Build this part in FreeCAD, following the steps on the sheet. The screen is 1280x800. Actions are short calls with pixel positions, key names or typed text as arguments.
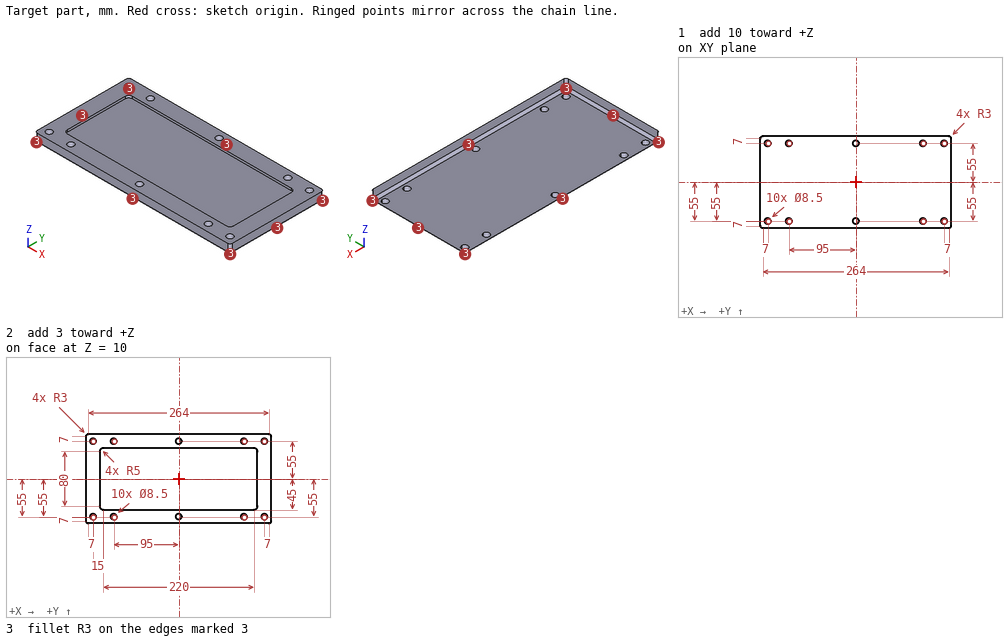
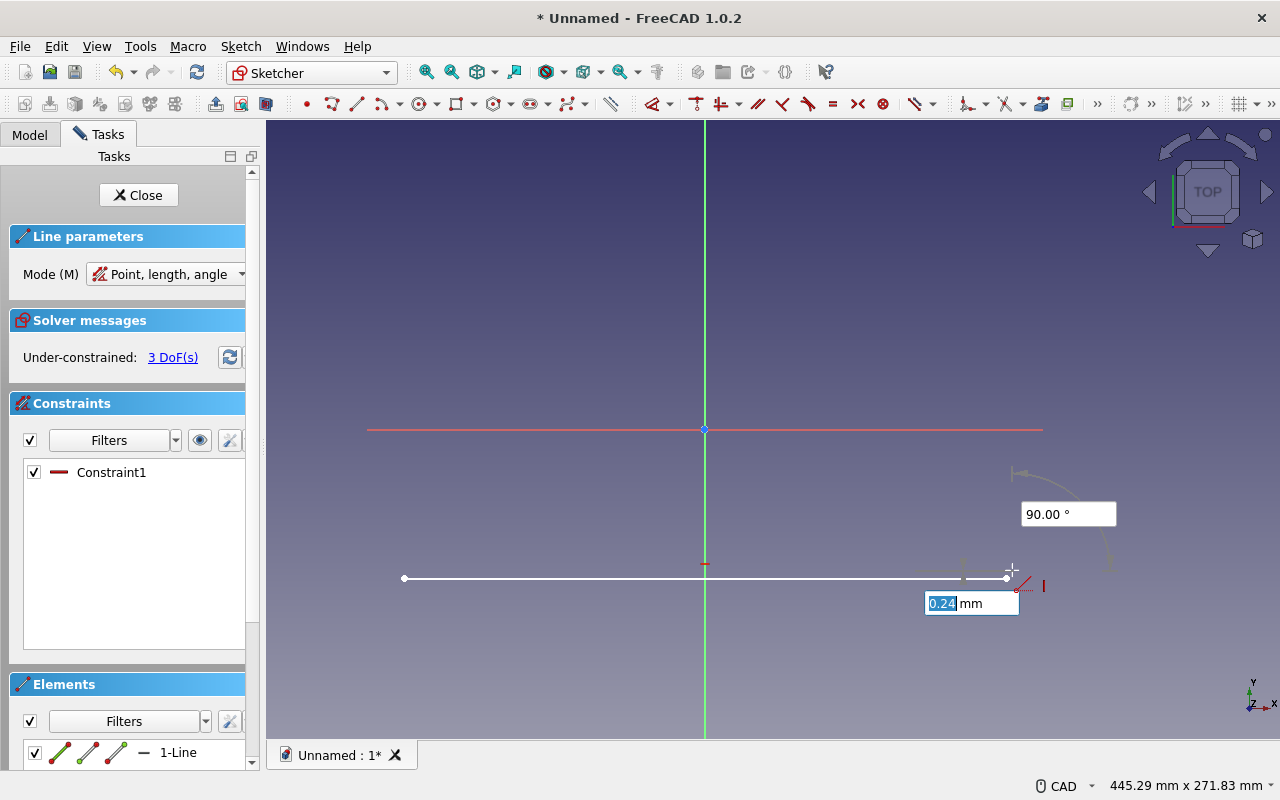
click(1012, 288)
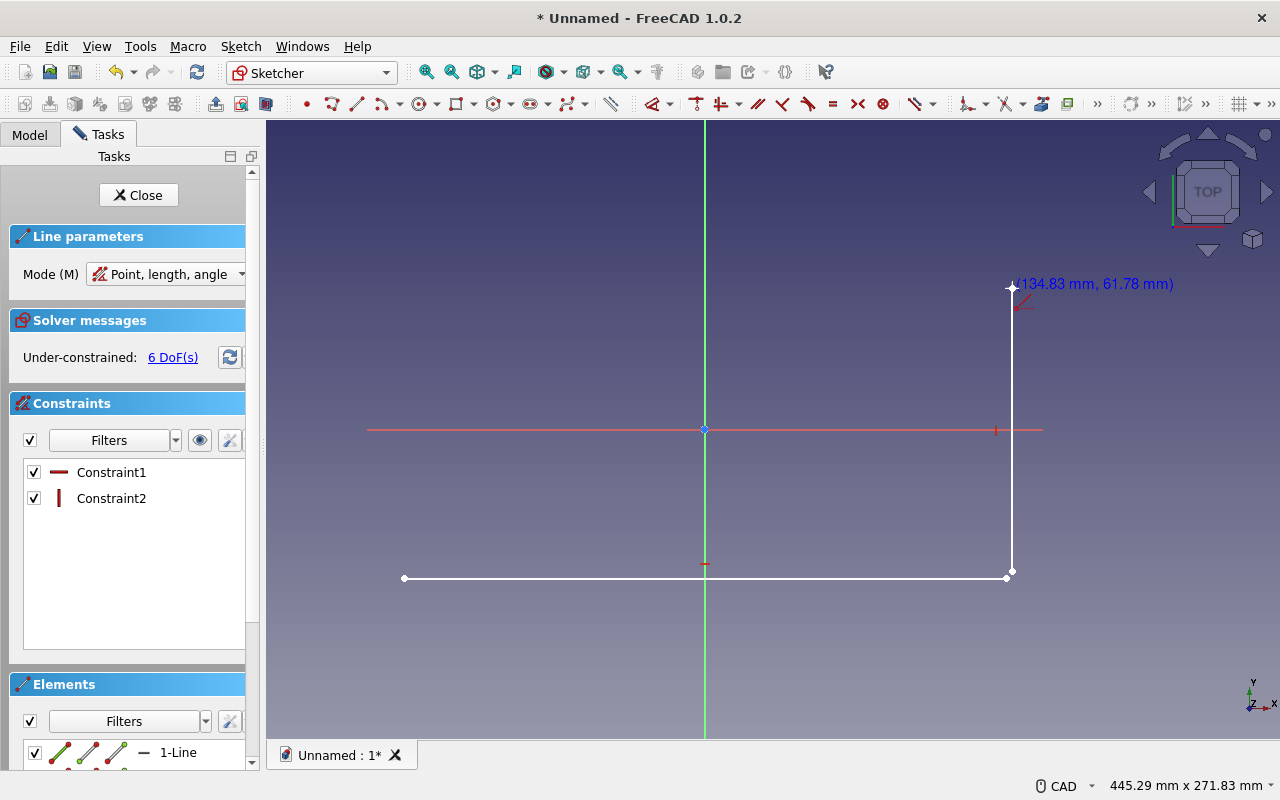
scroll(1006, 282, up, 3)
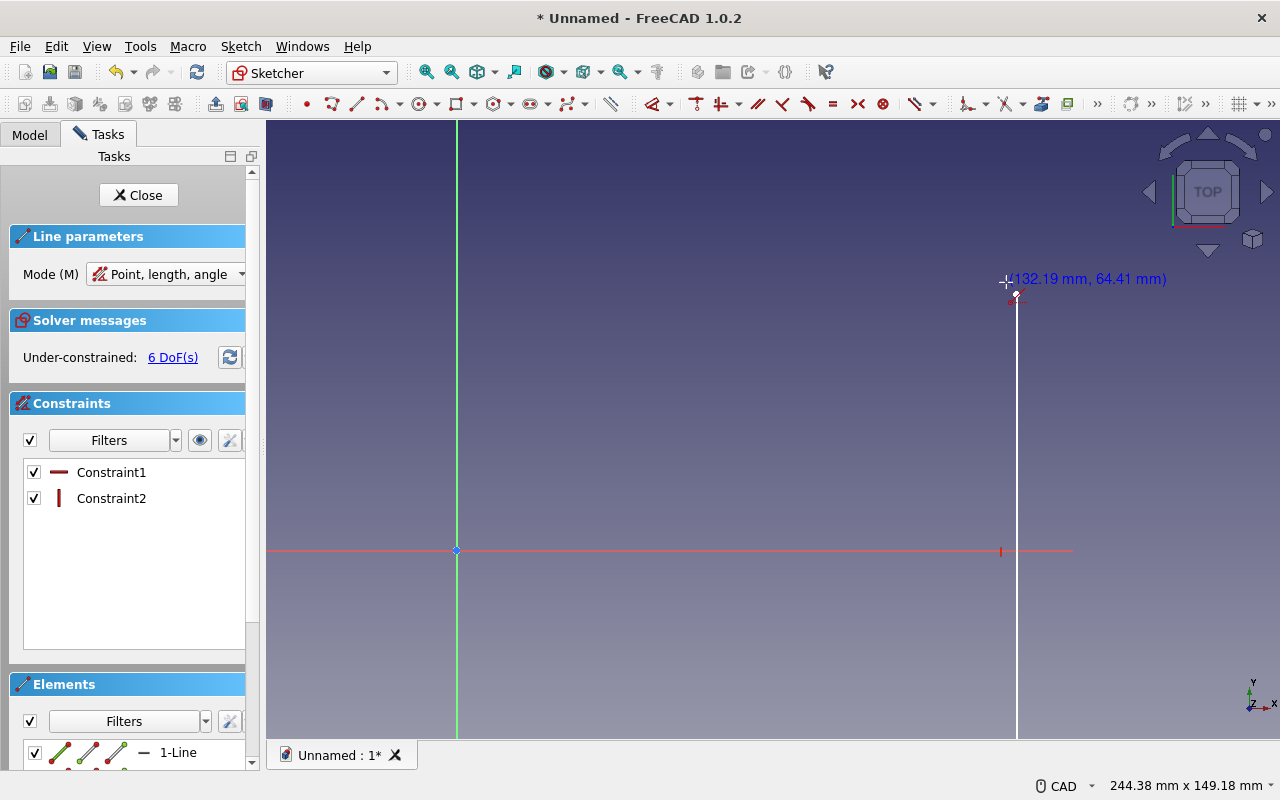
click(1005, 281)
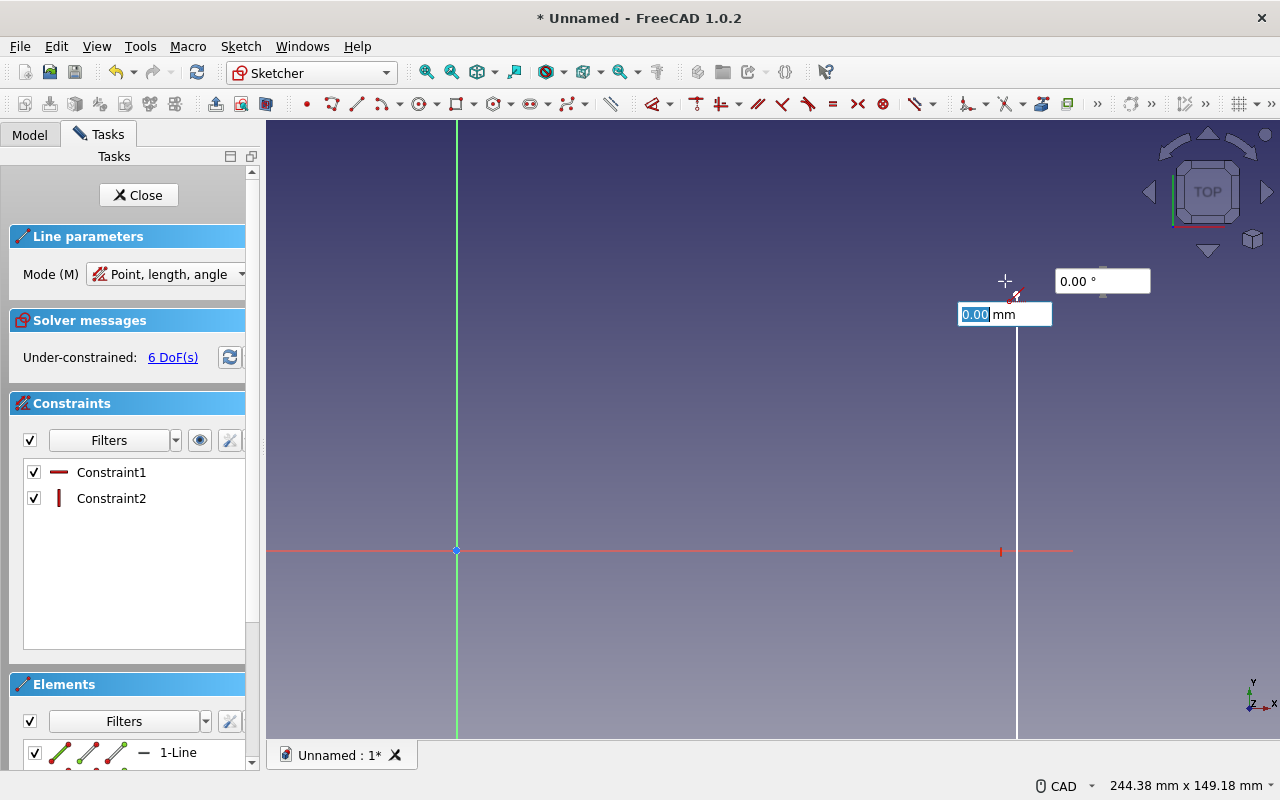
scroll(1006, 282, down, 3)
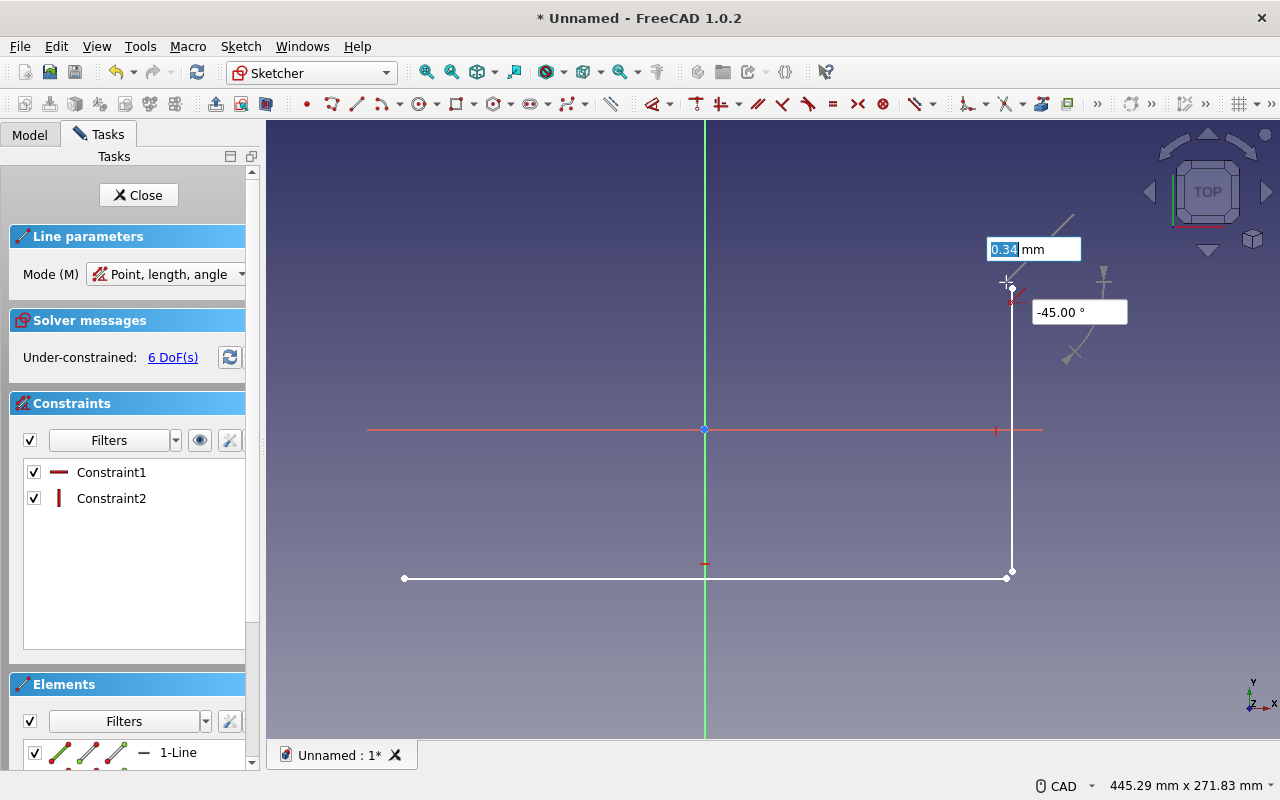
click(404, 282)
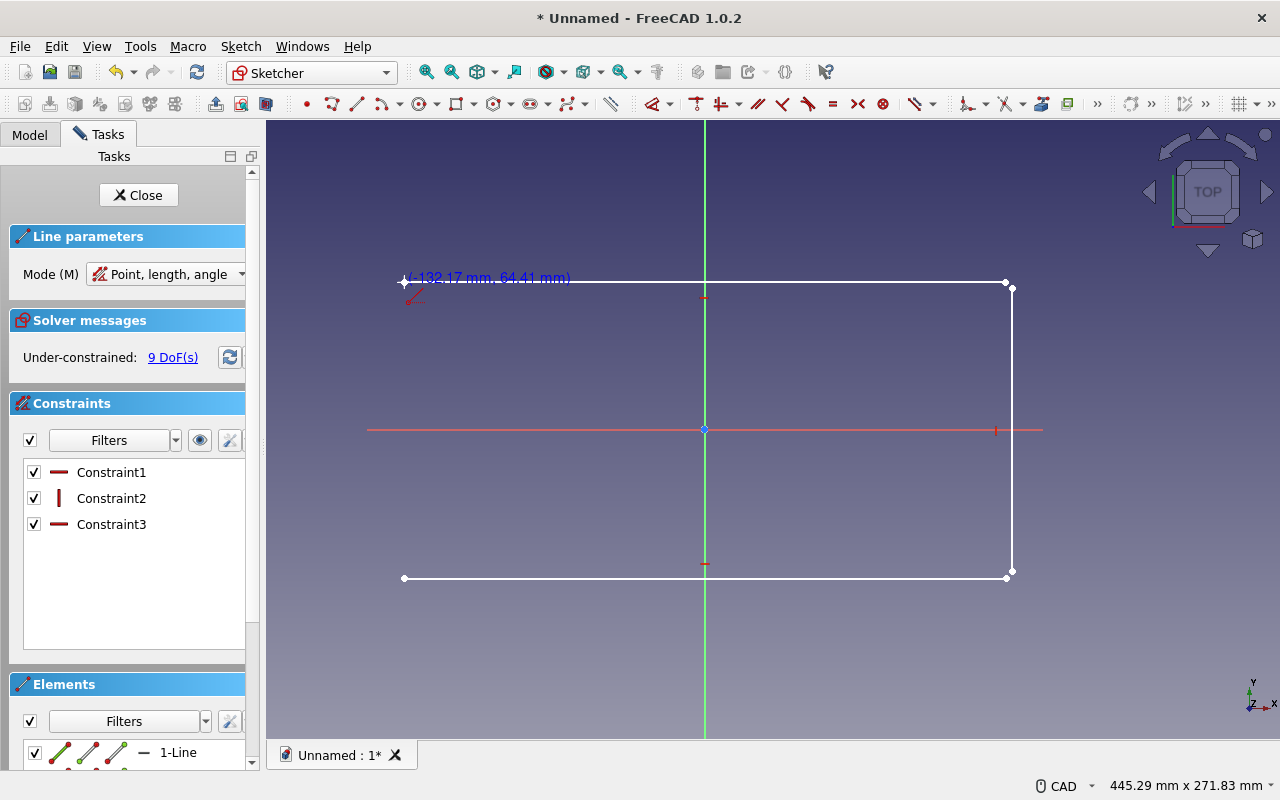
scroll(398, 288, up, 3)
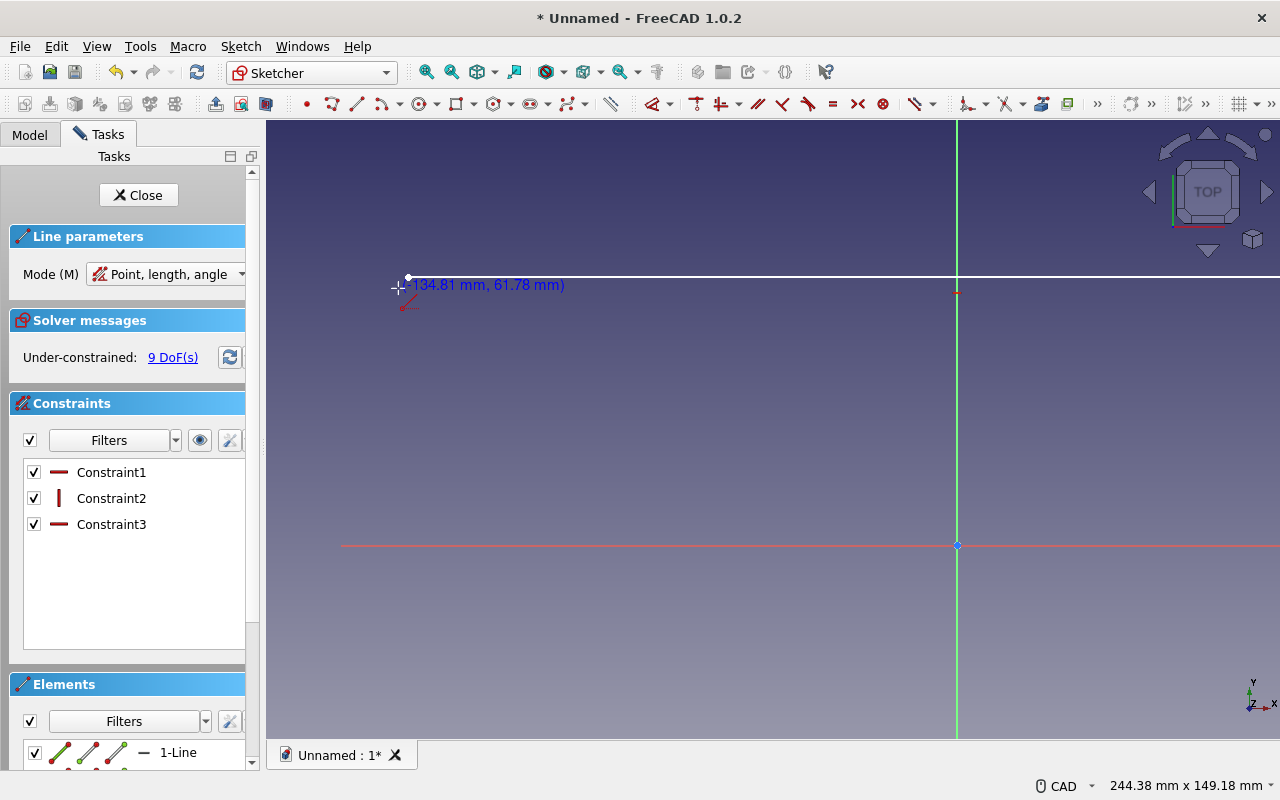
click(397, 289)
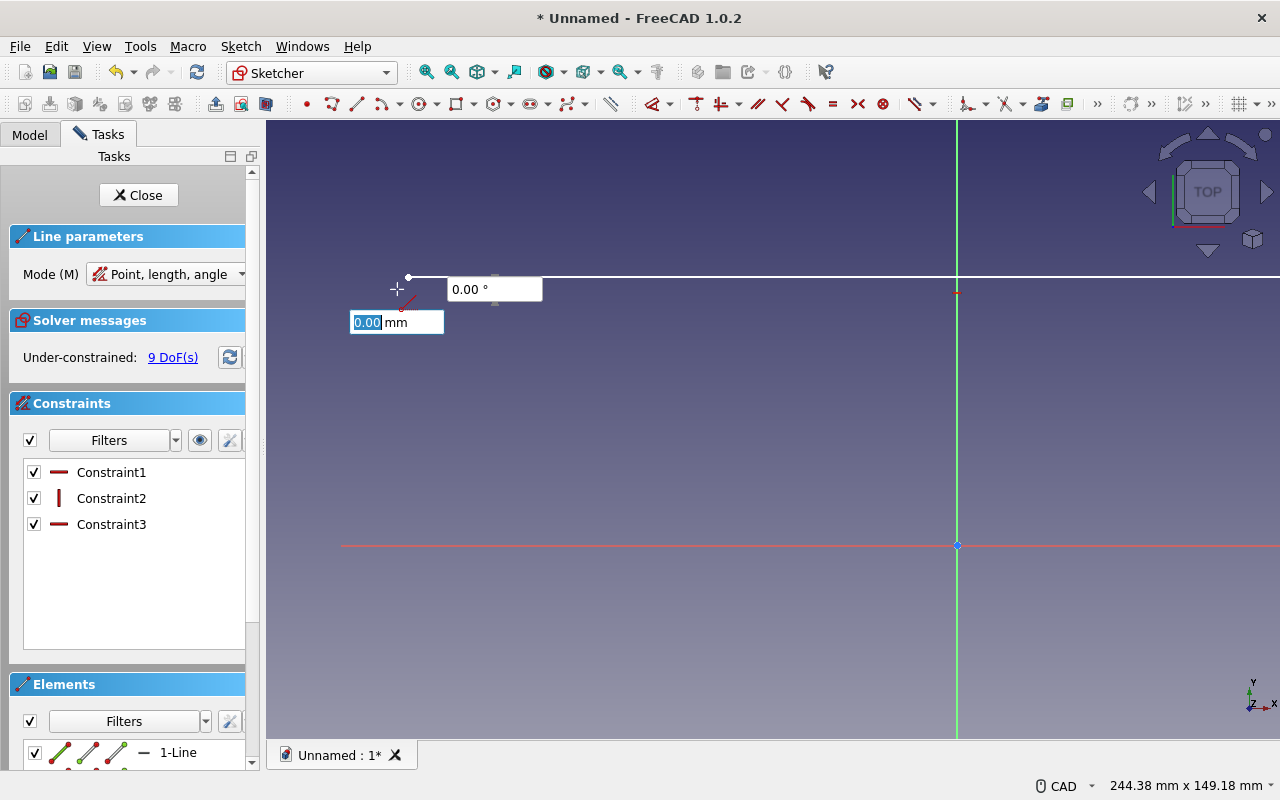
scroll(397, 288, down, 3)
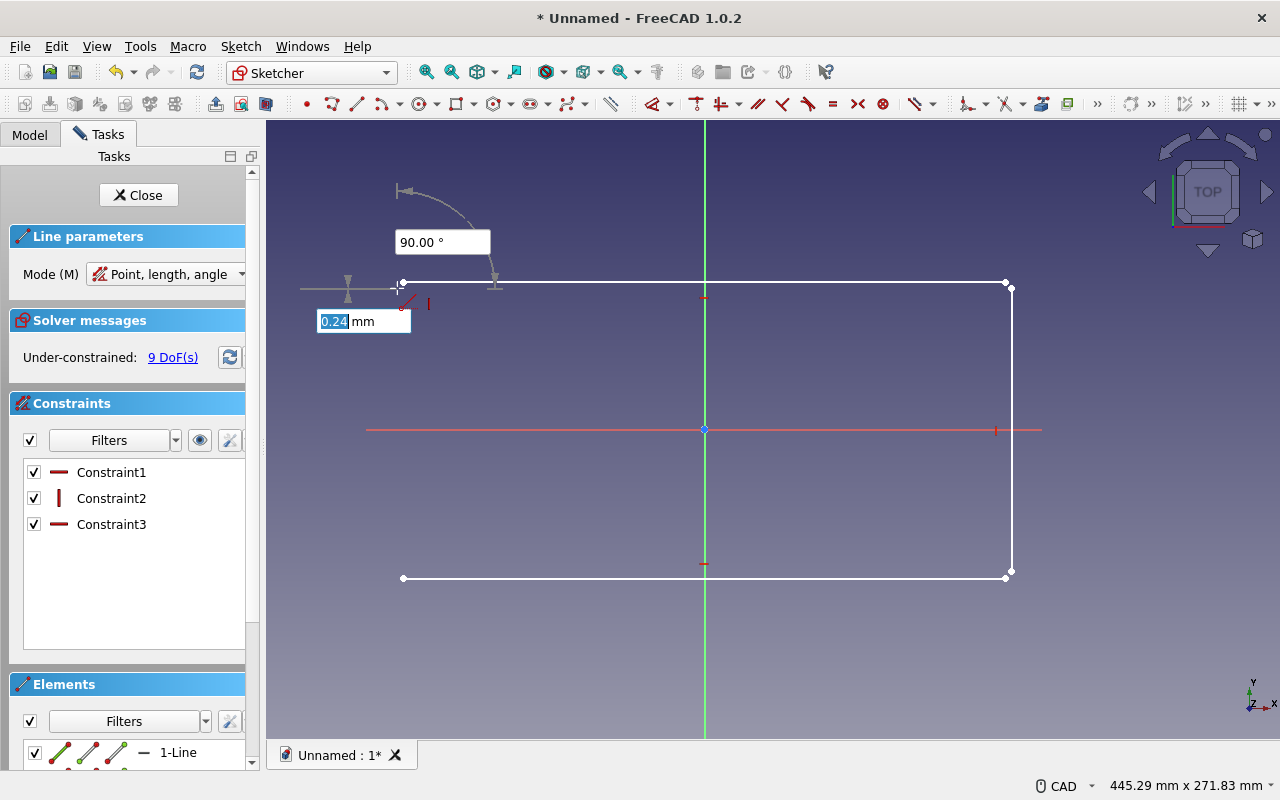
scroll(397, 571, up, 3)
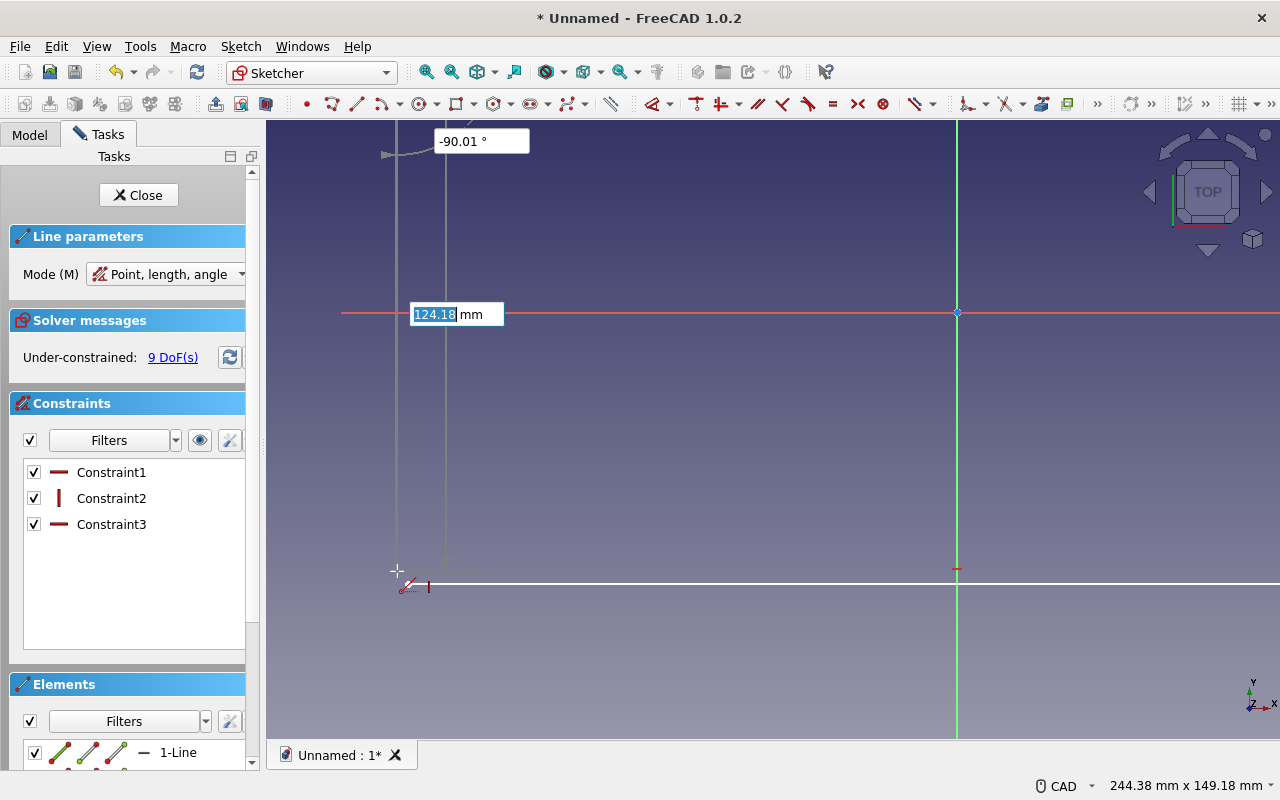
click(397, 570)